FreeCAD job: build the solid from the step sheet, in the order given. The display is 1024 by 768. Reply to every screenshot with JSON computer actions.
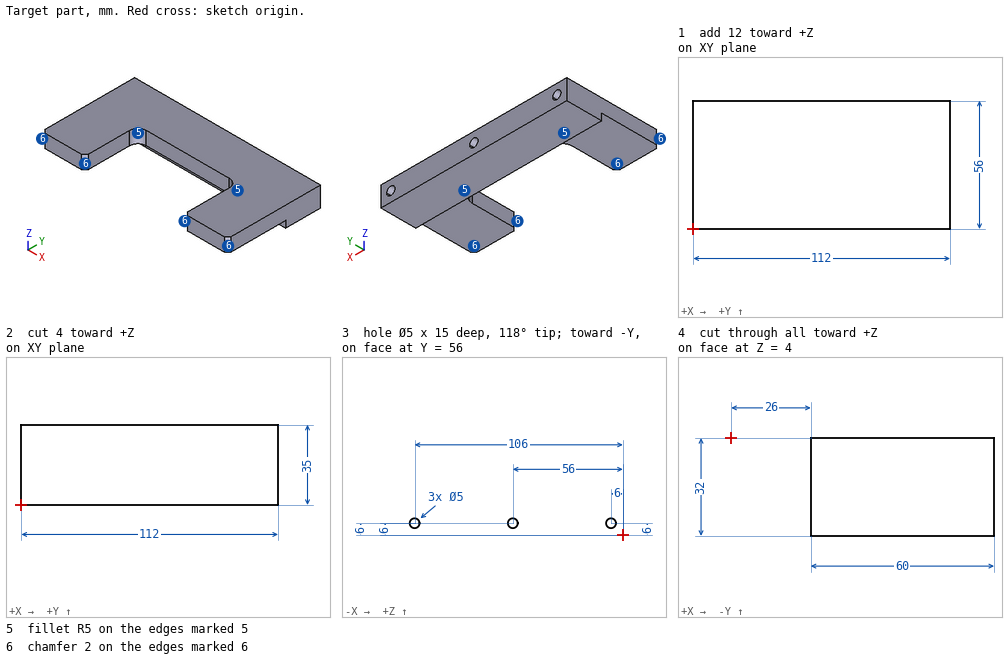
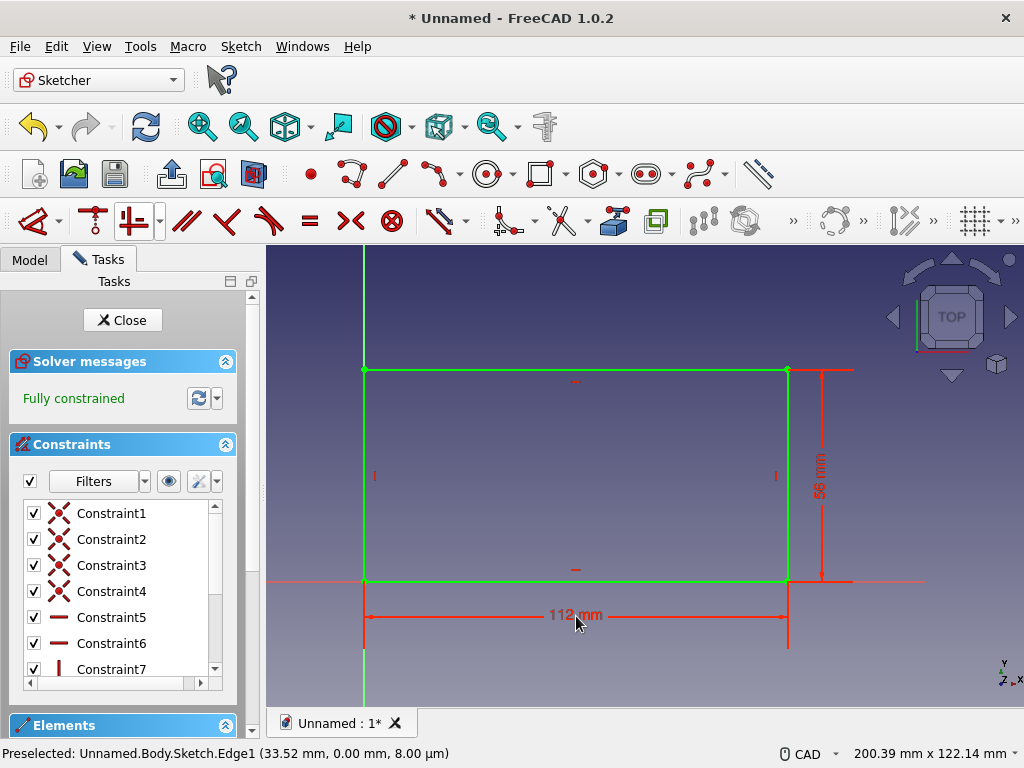
{"action": "left_click", "coordinate": [123, 320]}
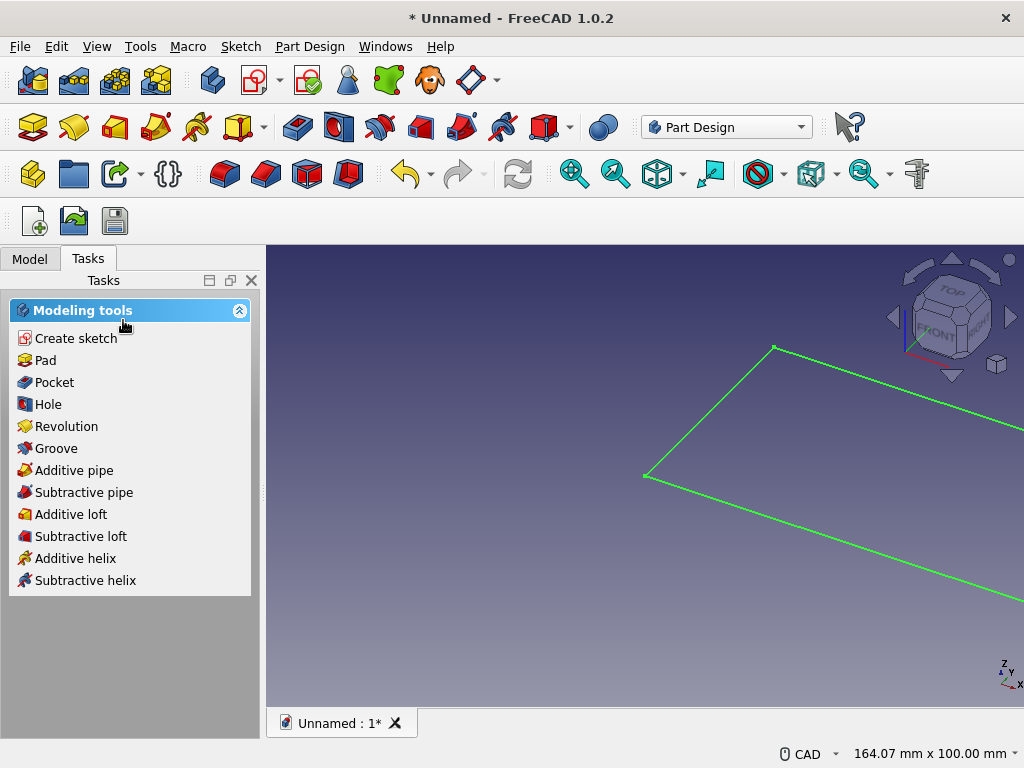
{"action": "left_click", "coordinate": [33, 128]}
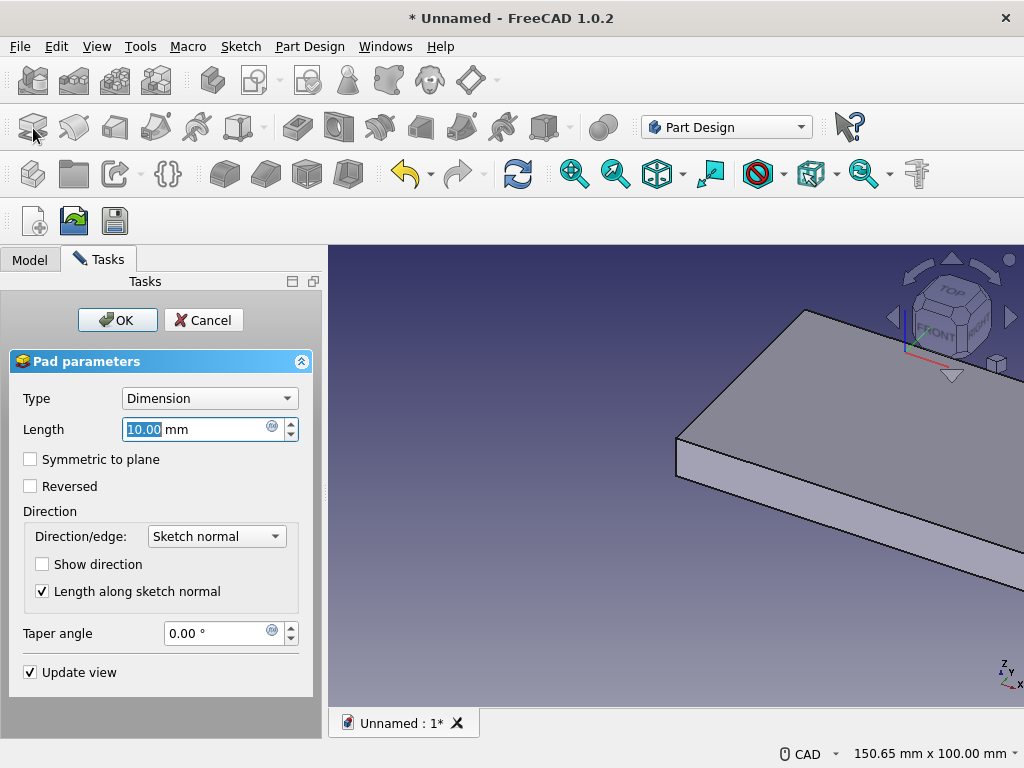
{"action": "type", "text": "12"}
{"action": "key", "text": "Tab"}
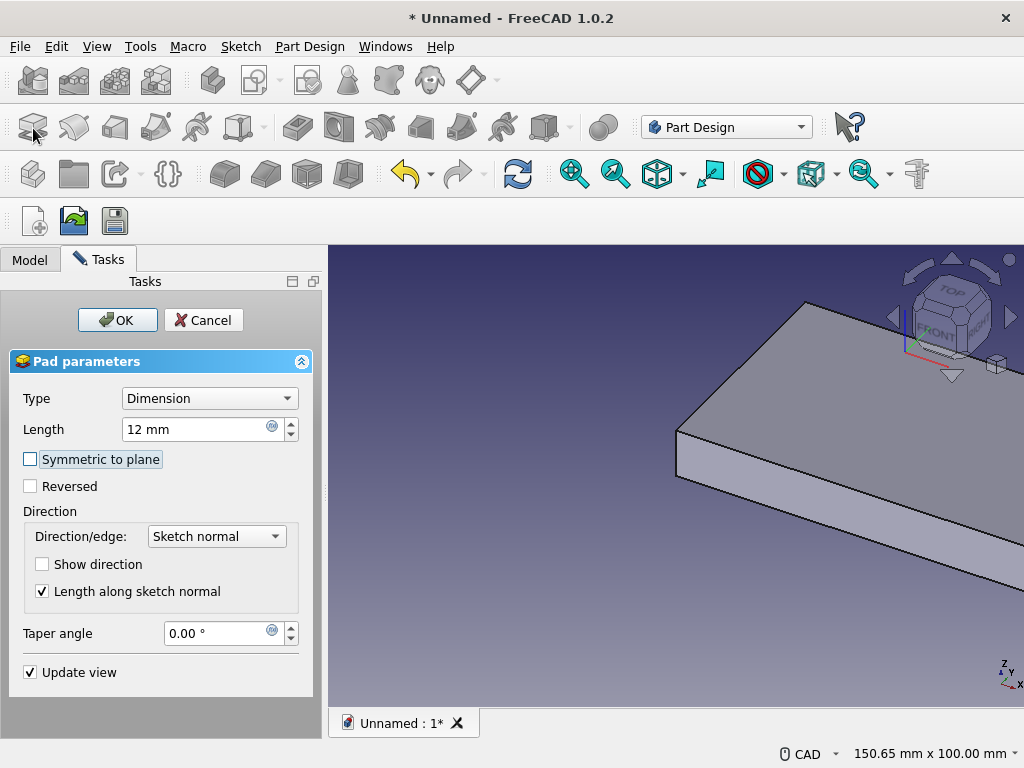
{"action": "left_click", "coordinate": [118, 320]}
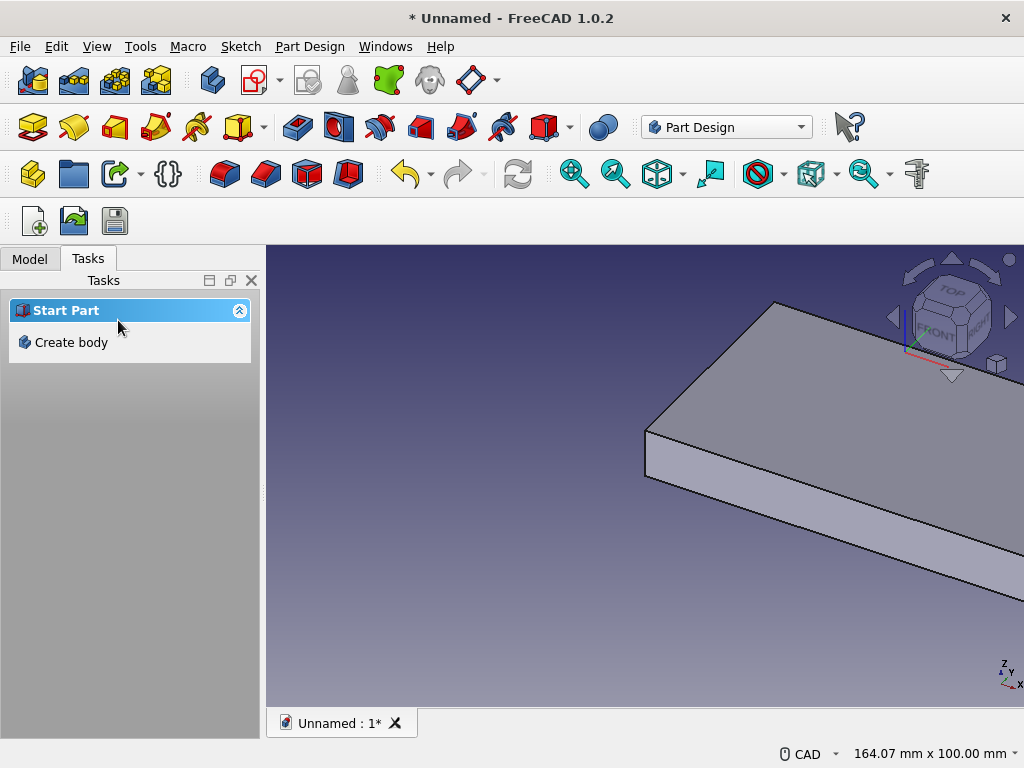
{"action": "left_click", "coordinate": [575, 174]}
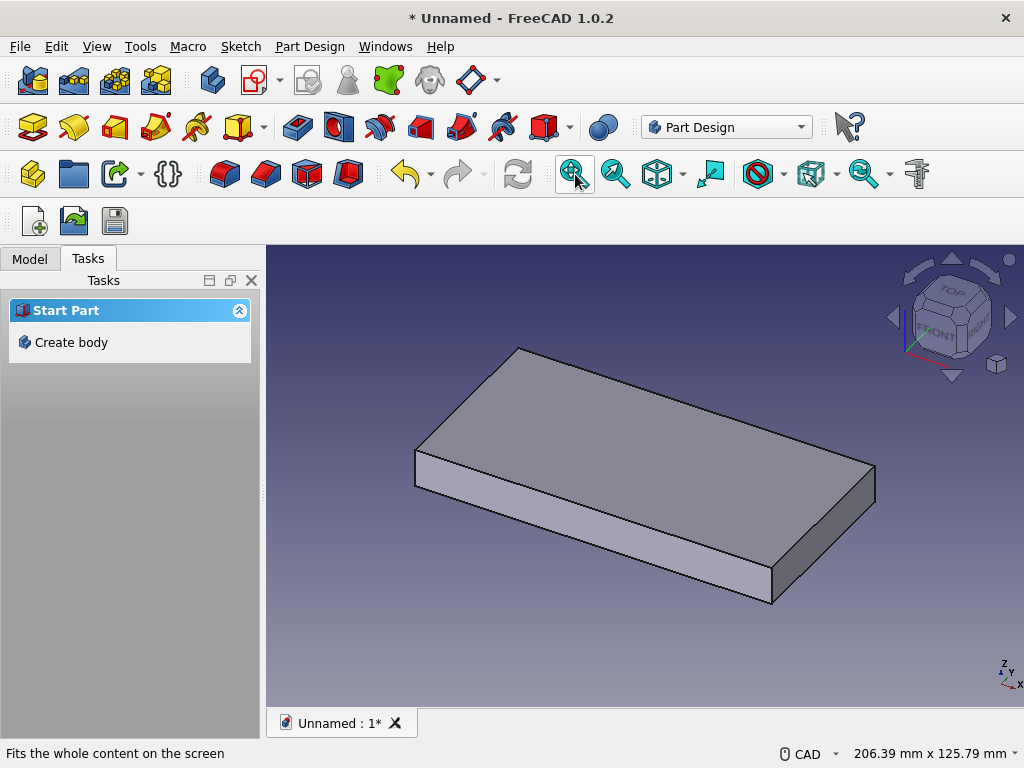
{"action": "left_click", "coordinate": [254, 80]}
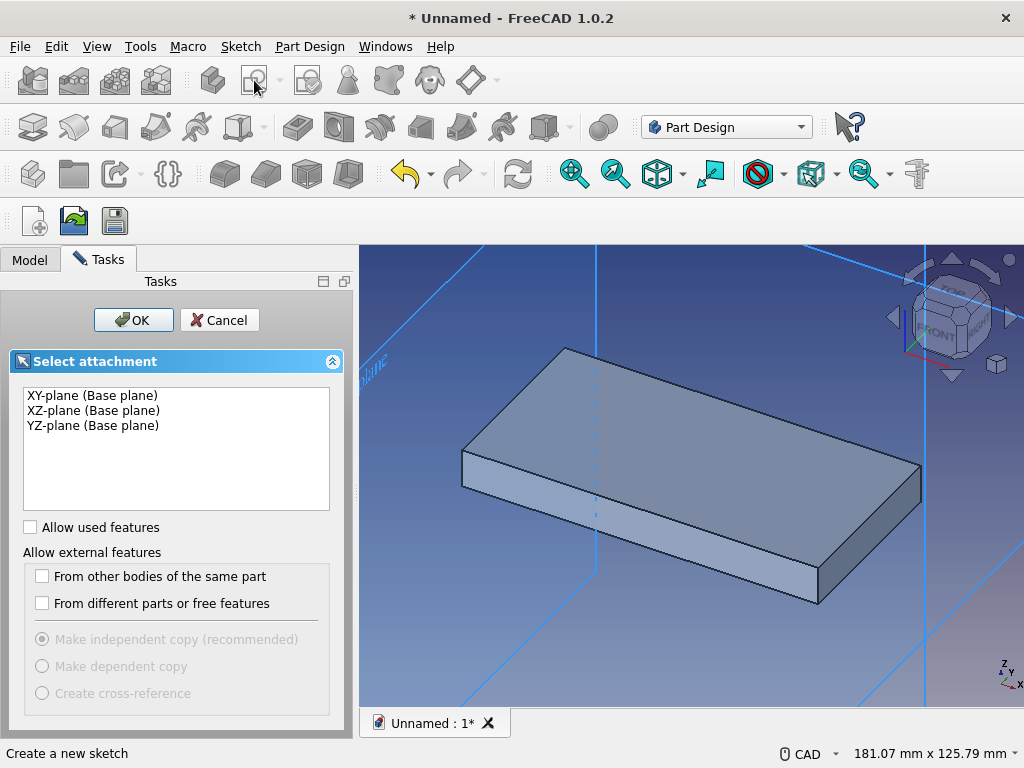
{"action": "left_click", "coordinate": [84, 396]}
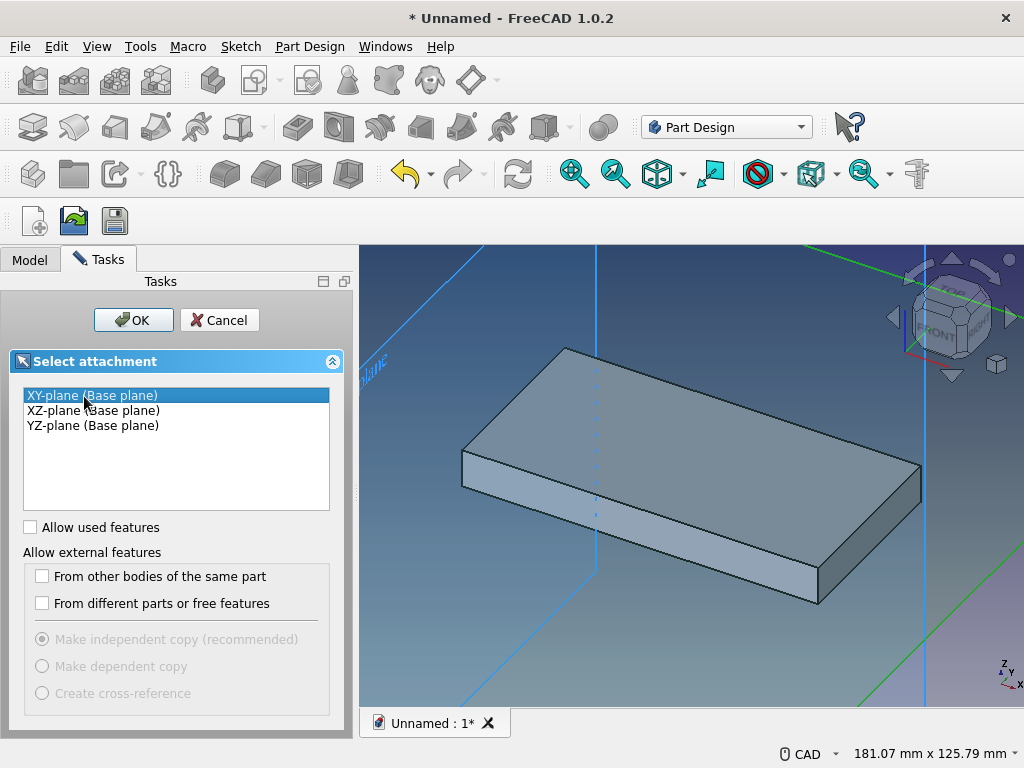
{"action": "left_click", "coordinate": [134, 320]}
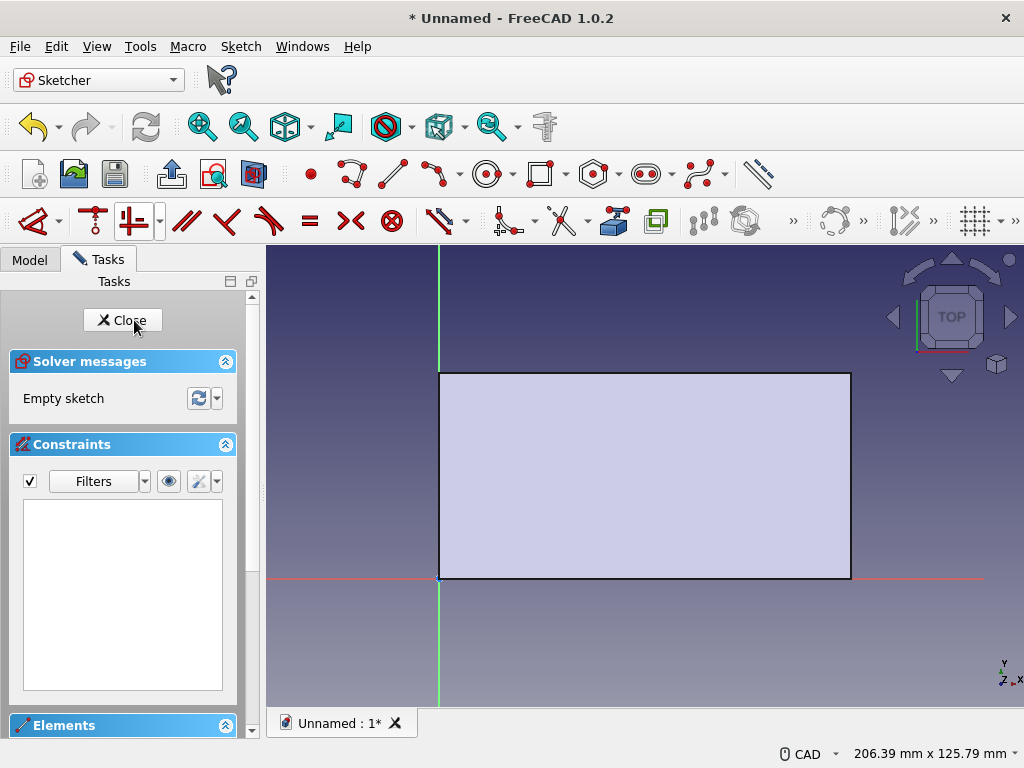
{"action": "key", "text": "q s"}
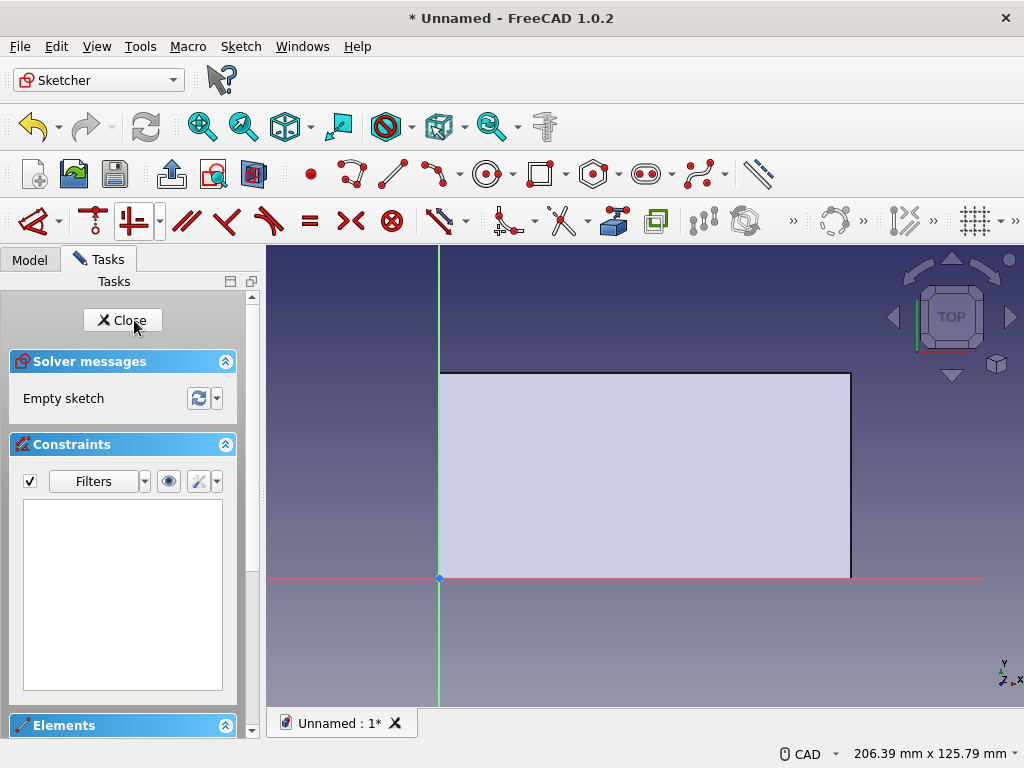
{"action": "scroll", "coordinate": [294, 302], "scroll_direction": "down", "scroll_amount": 1}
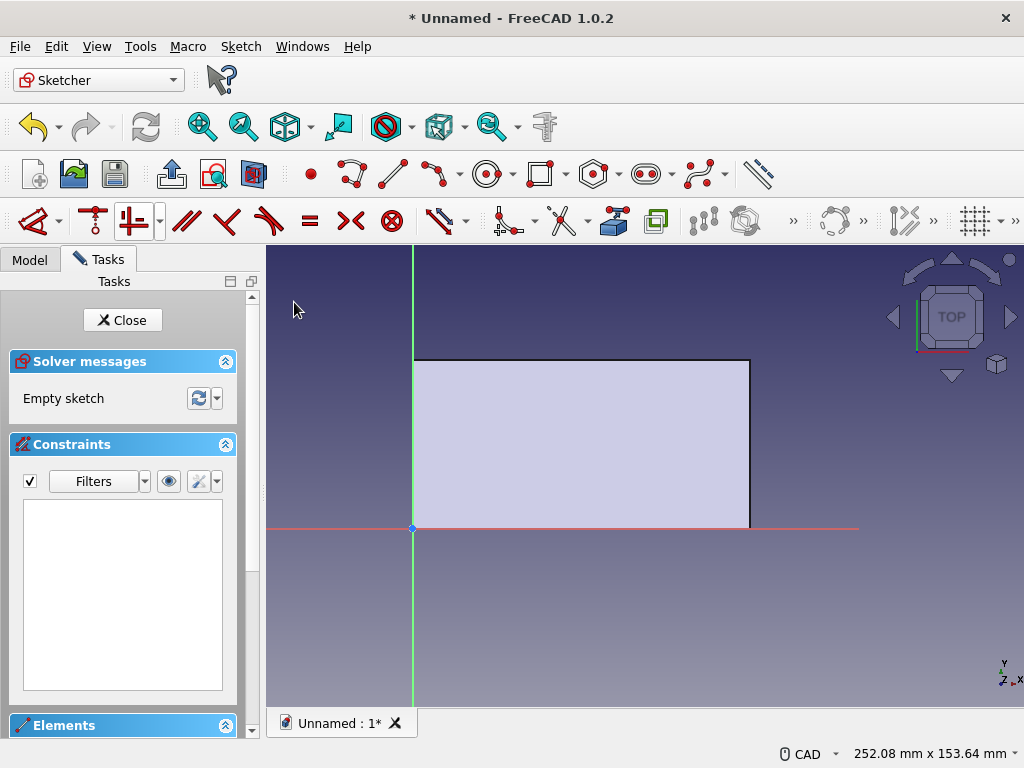
{"action": "left_click", "coordinate": [540, 174]}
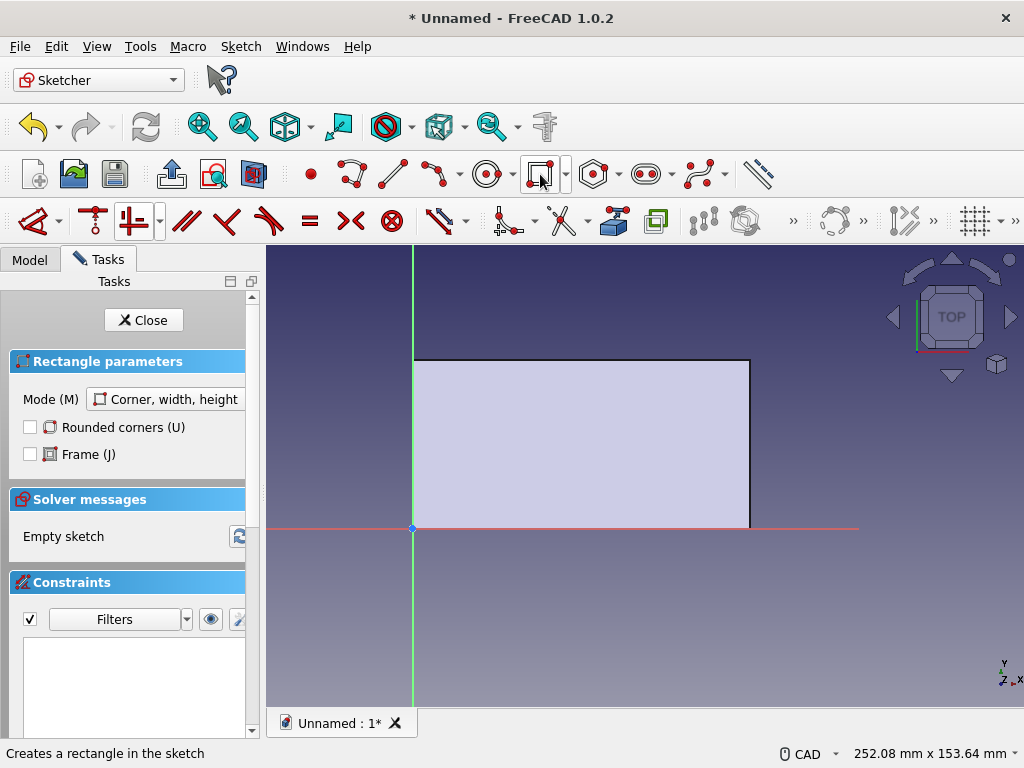
{"action": "left_click", "coordinate": [413, 529]}
{"action": "left_click", "coordinate": [750, 423]}
{"action": "key", "text": "Escape"}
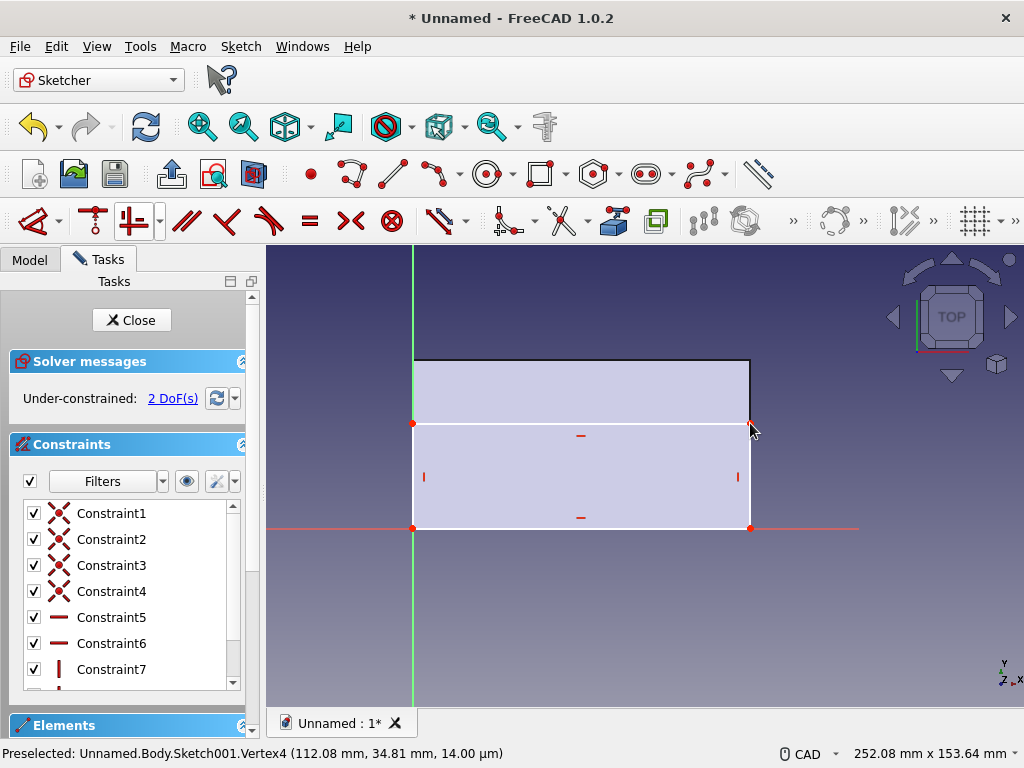
{"action": "left_click", "coordinate": [32, 222]}